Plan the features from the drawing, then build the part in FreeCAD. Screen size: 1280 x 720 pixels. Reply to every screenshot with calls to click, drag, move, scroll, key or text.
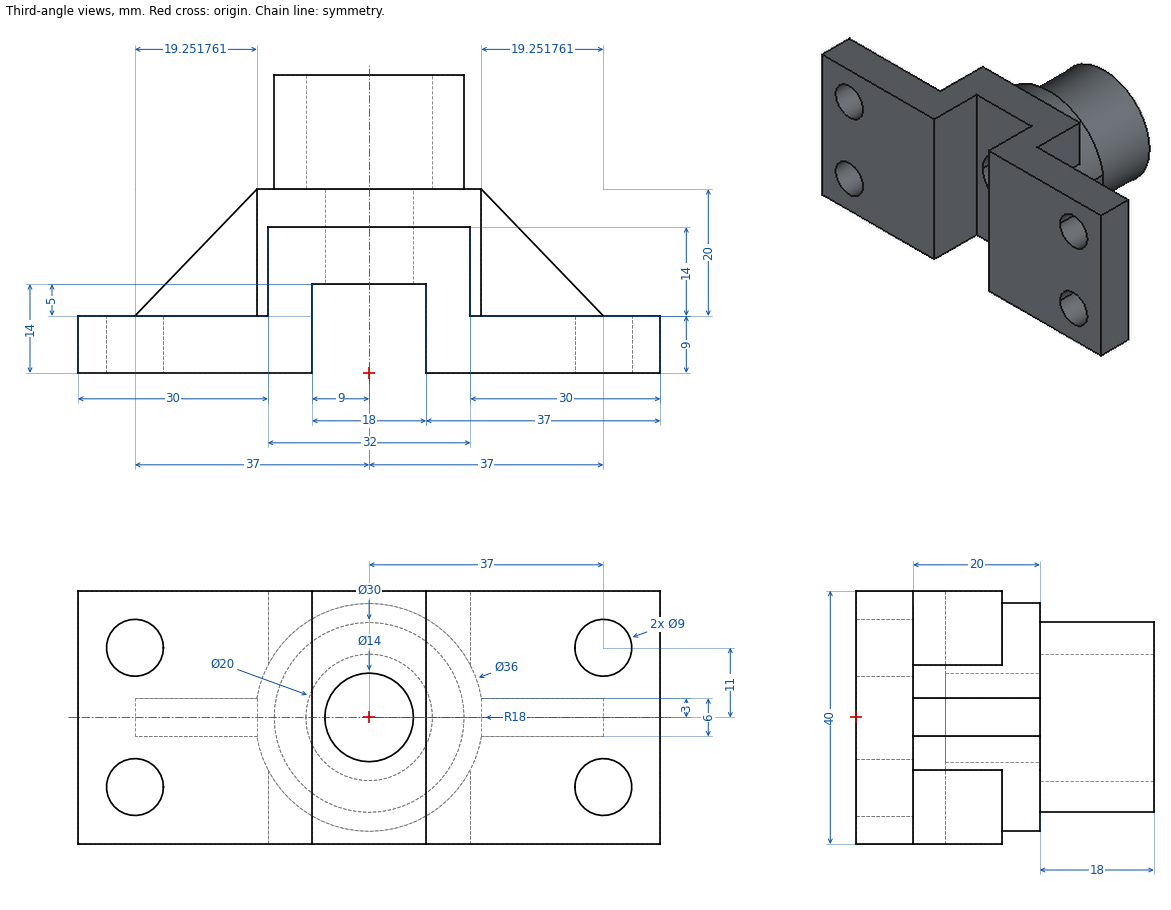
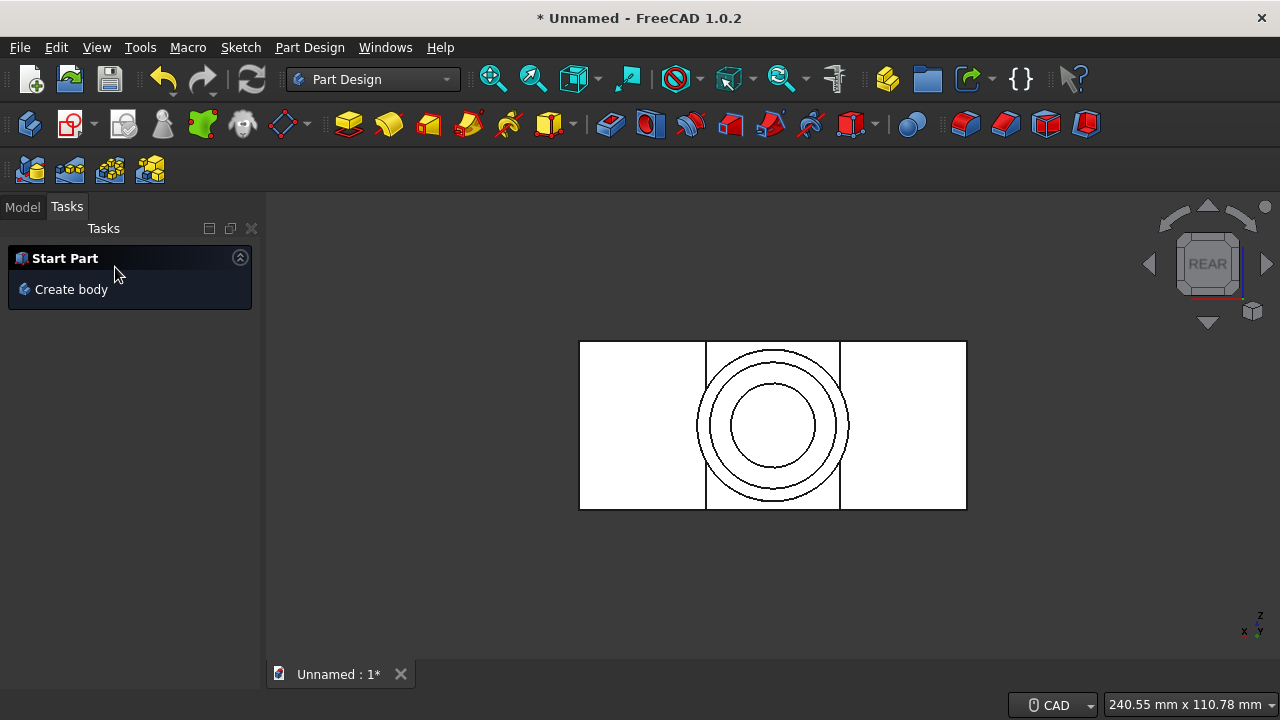
click(494, 80)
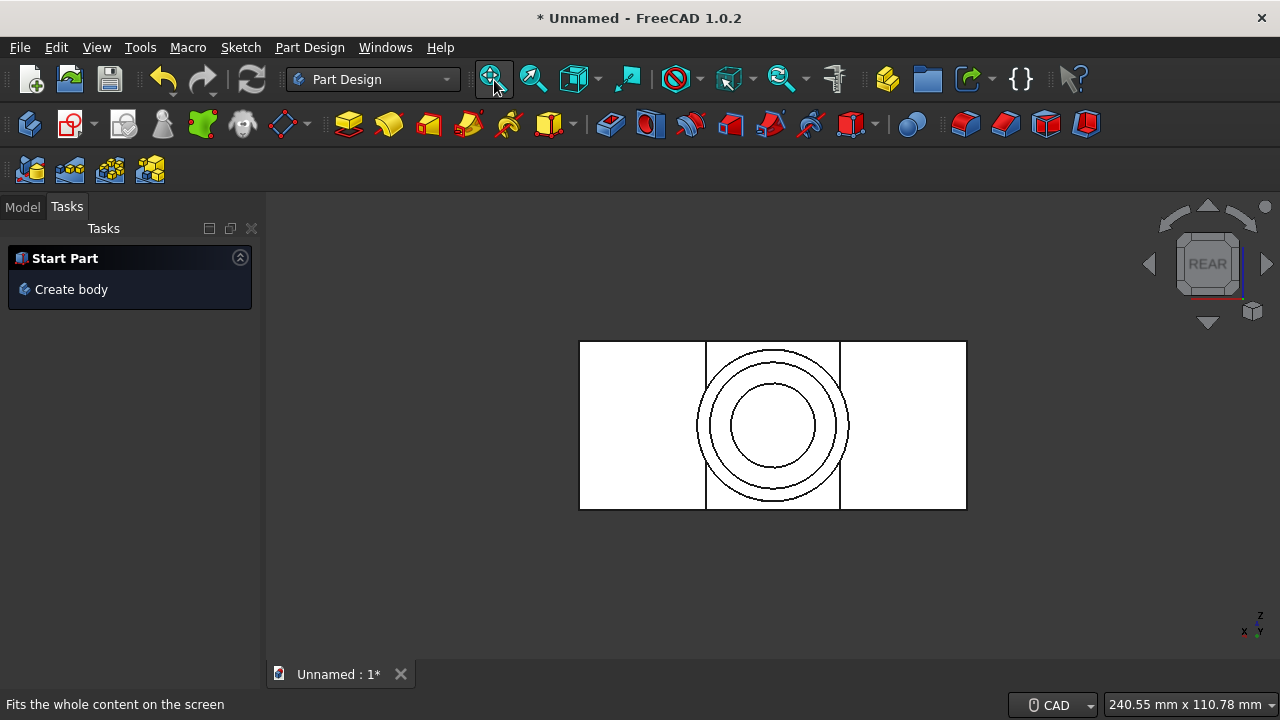
click(773, 424)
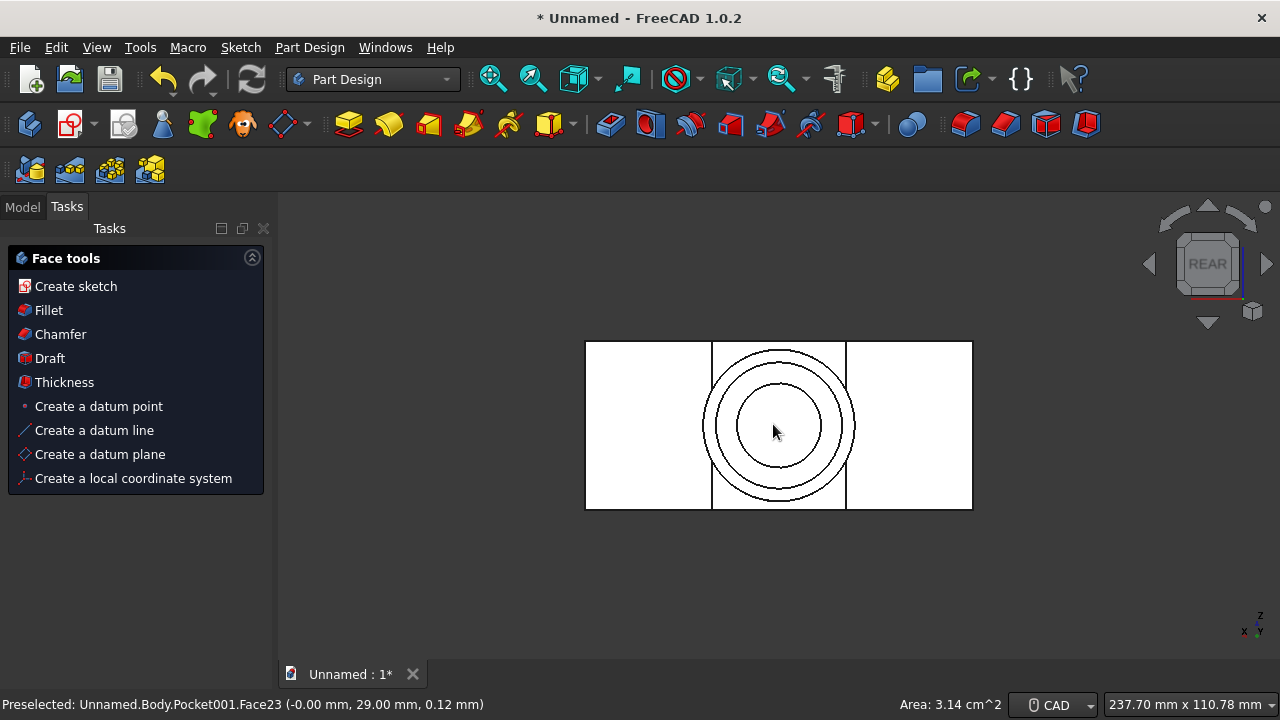
click(70, 124)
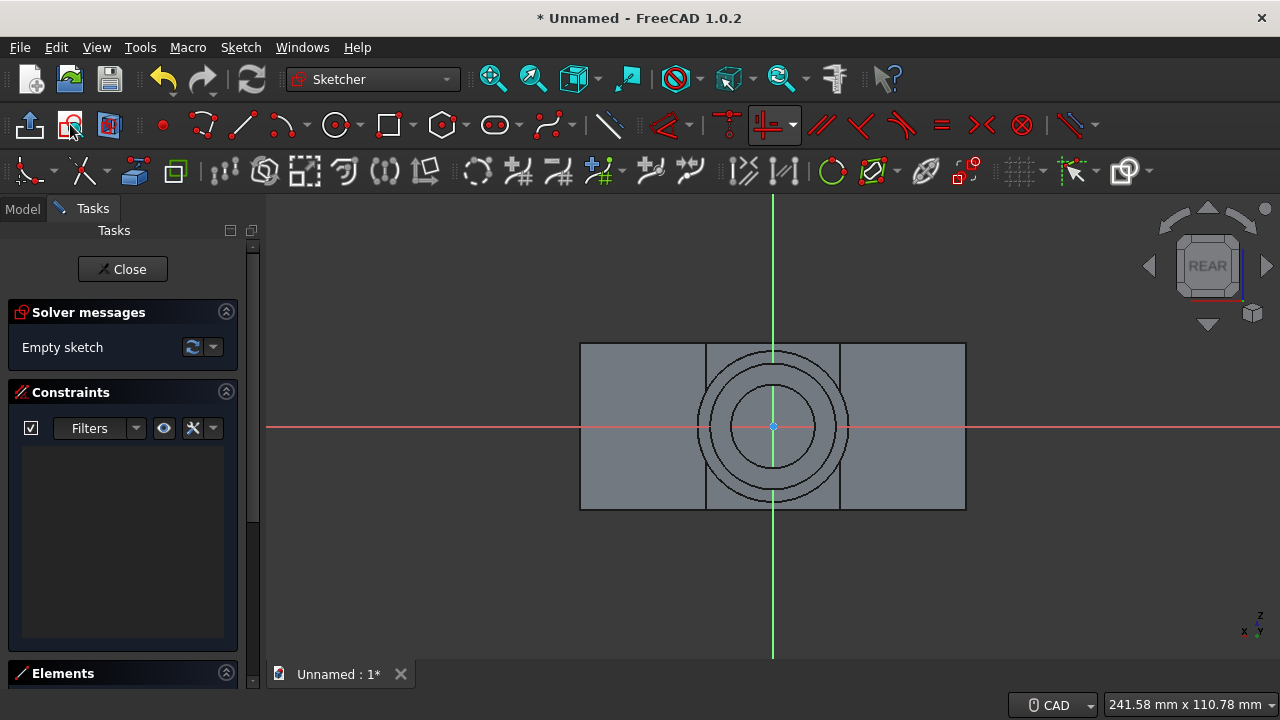
key(q)
key(s)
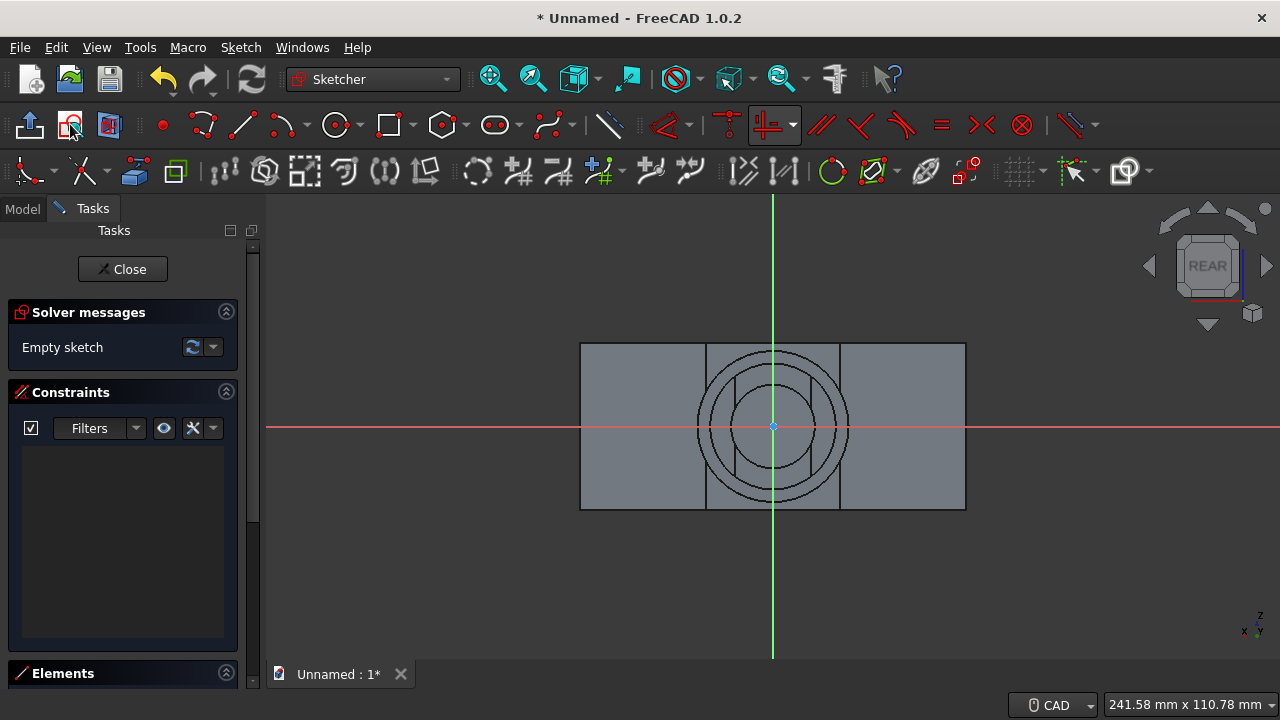
scroll(790, 426, up, 8)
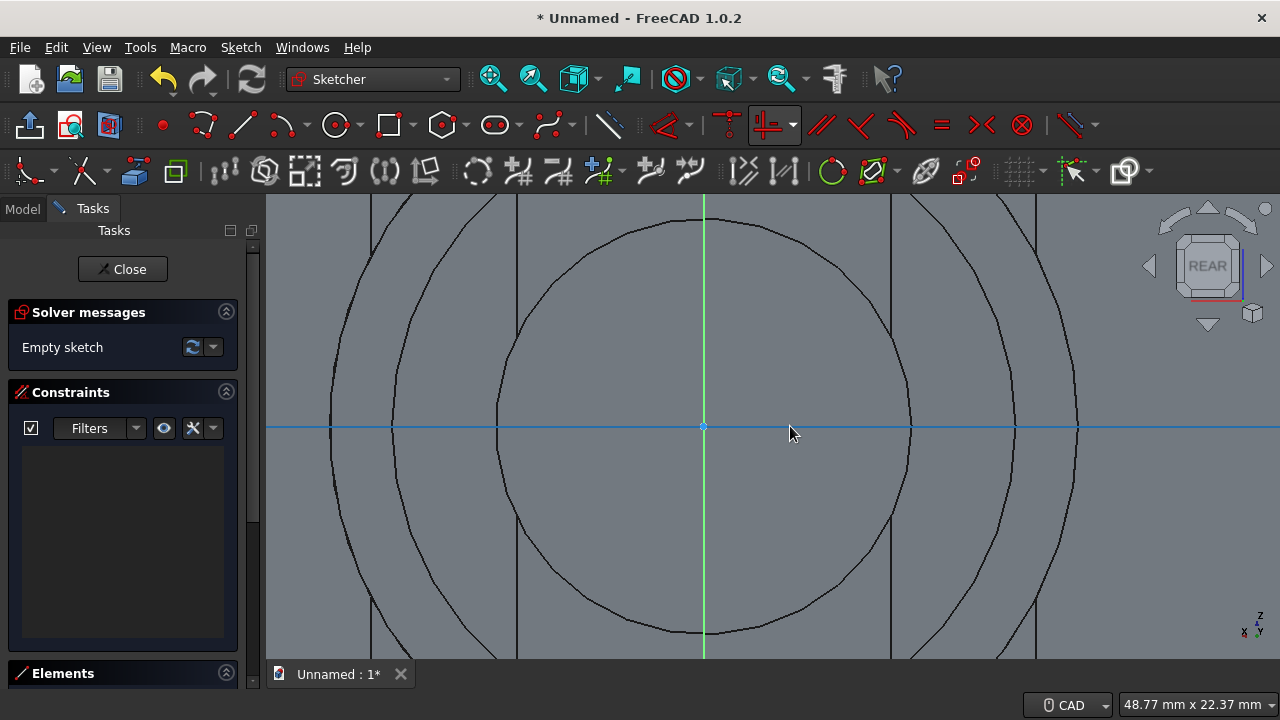
key(g)
key(c)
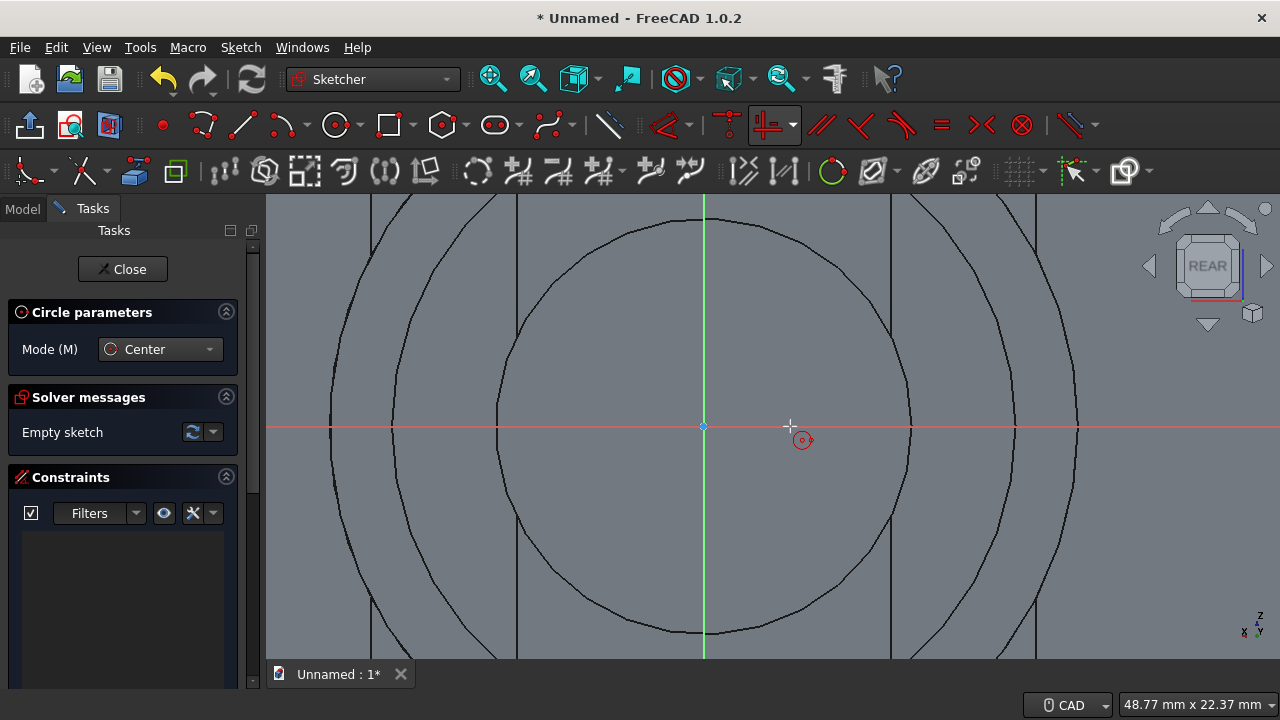
click(704, 426)
click(807, 324)
key(Escape)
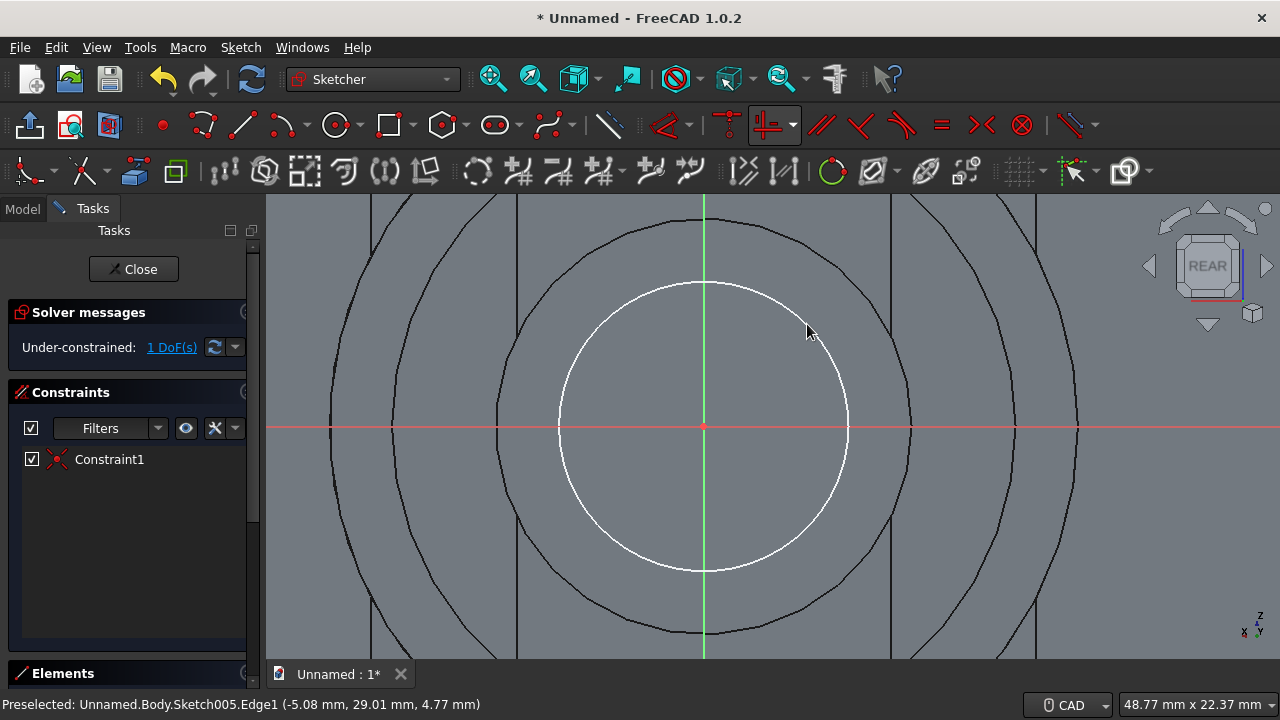
click(664, 126)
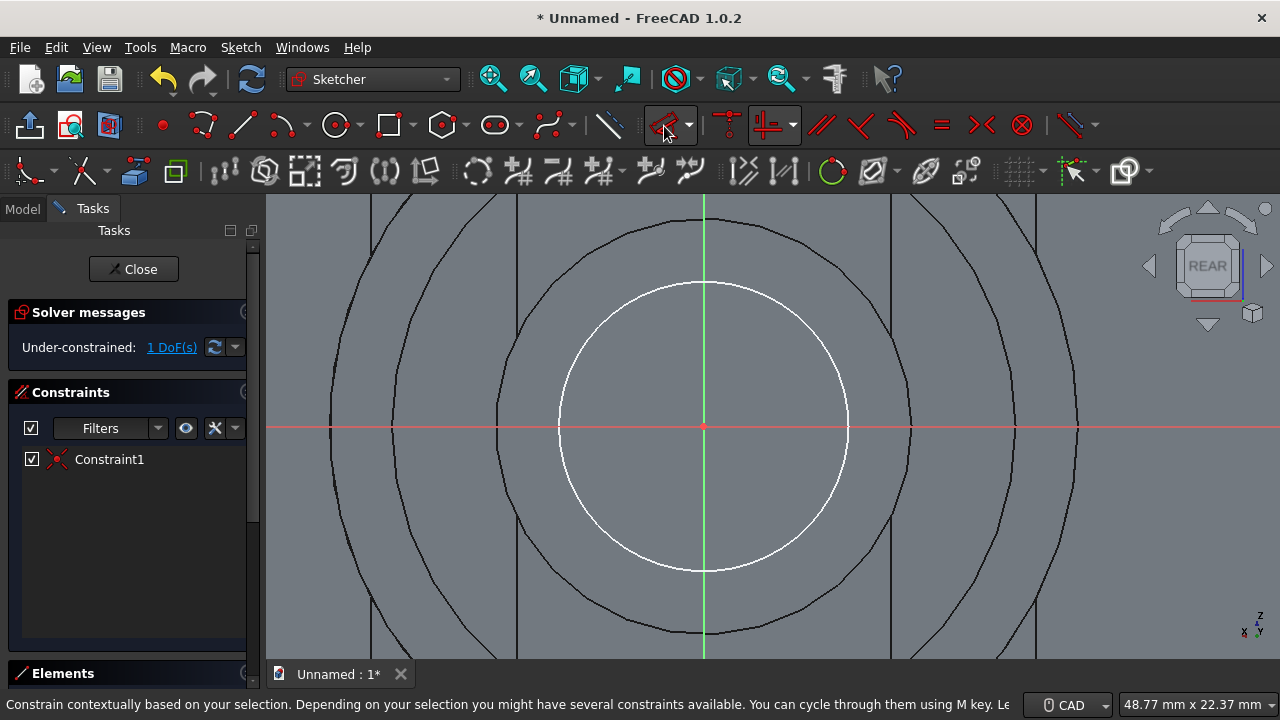
click(806, 324)
click(829, 301)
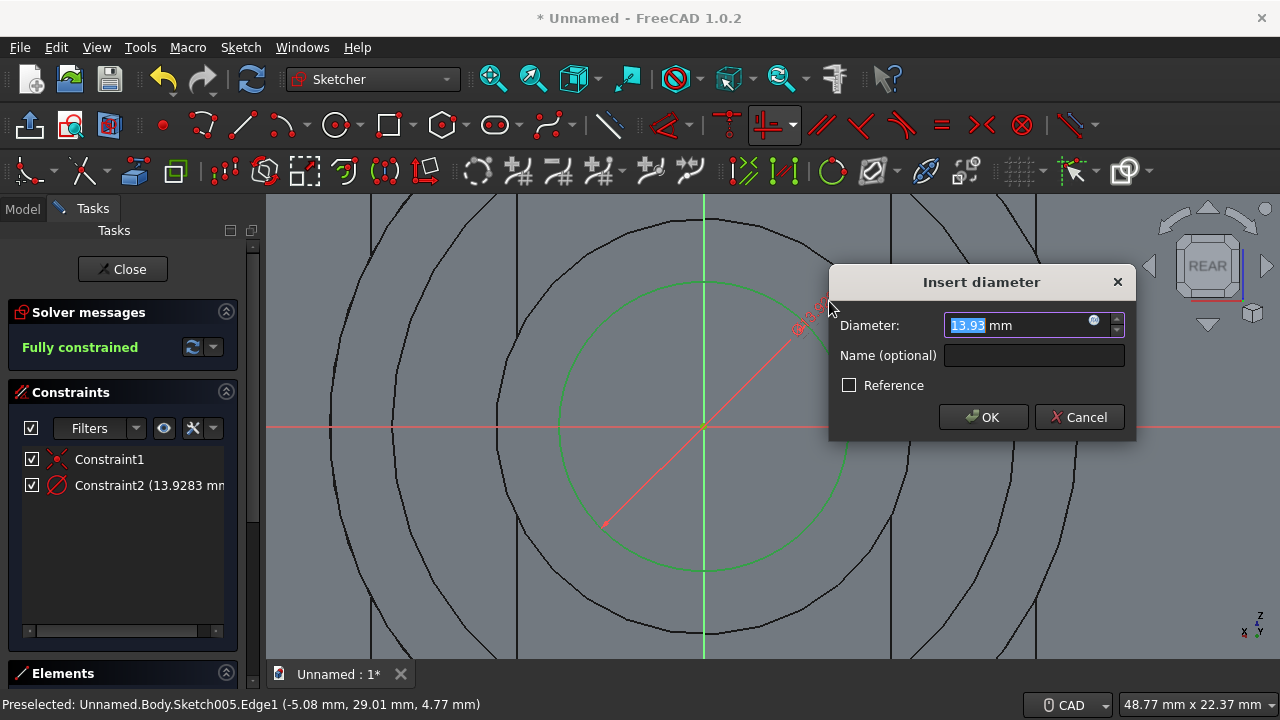
text(14)
key(Return)
key(Escape)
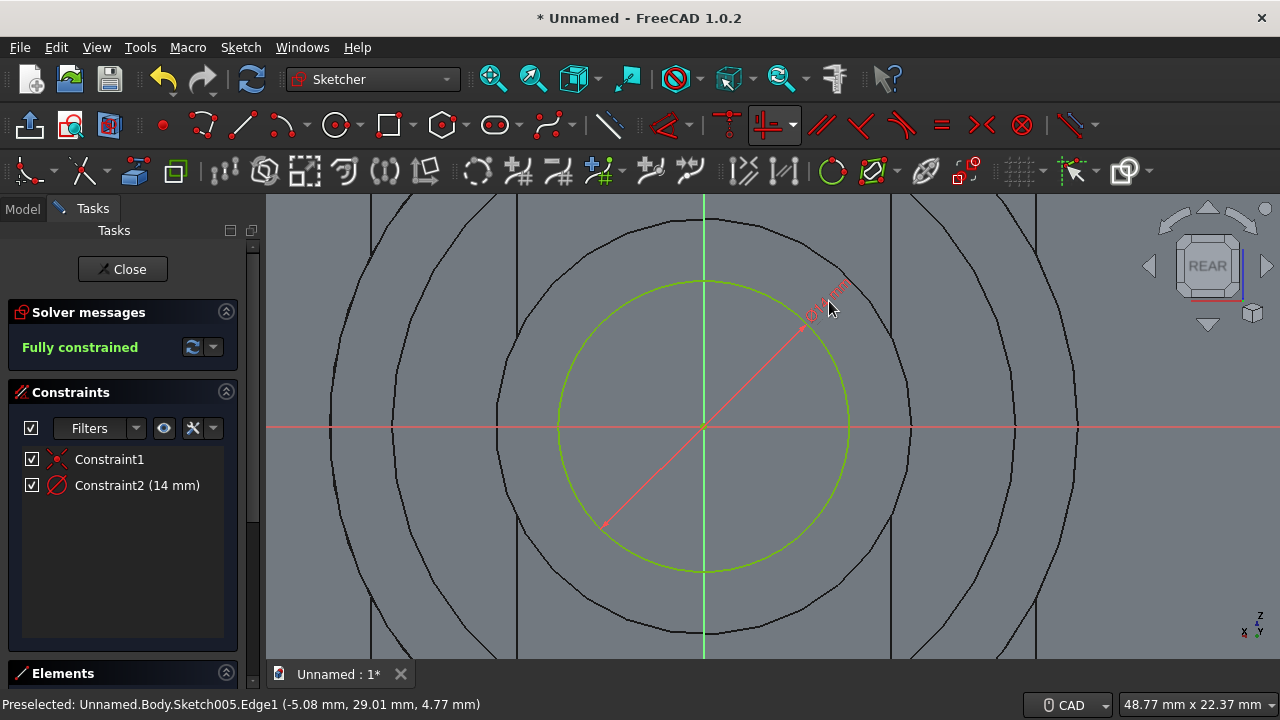
click(123, 269)